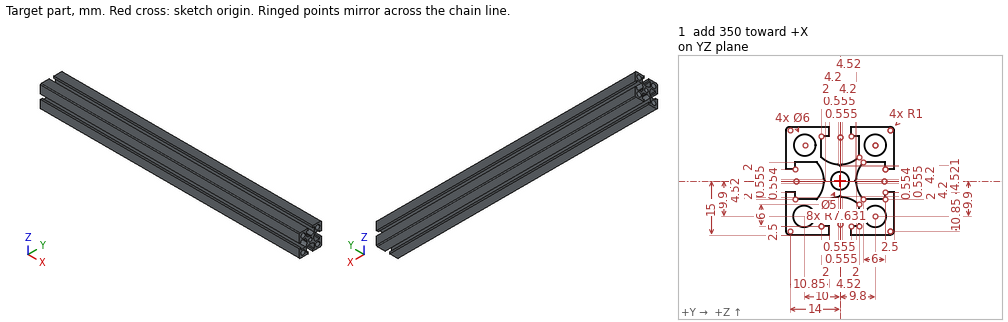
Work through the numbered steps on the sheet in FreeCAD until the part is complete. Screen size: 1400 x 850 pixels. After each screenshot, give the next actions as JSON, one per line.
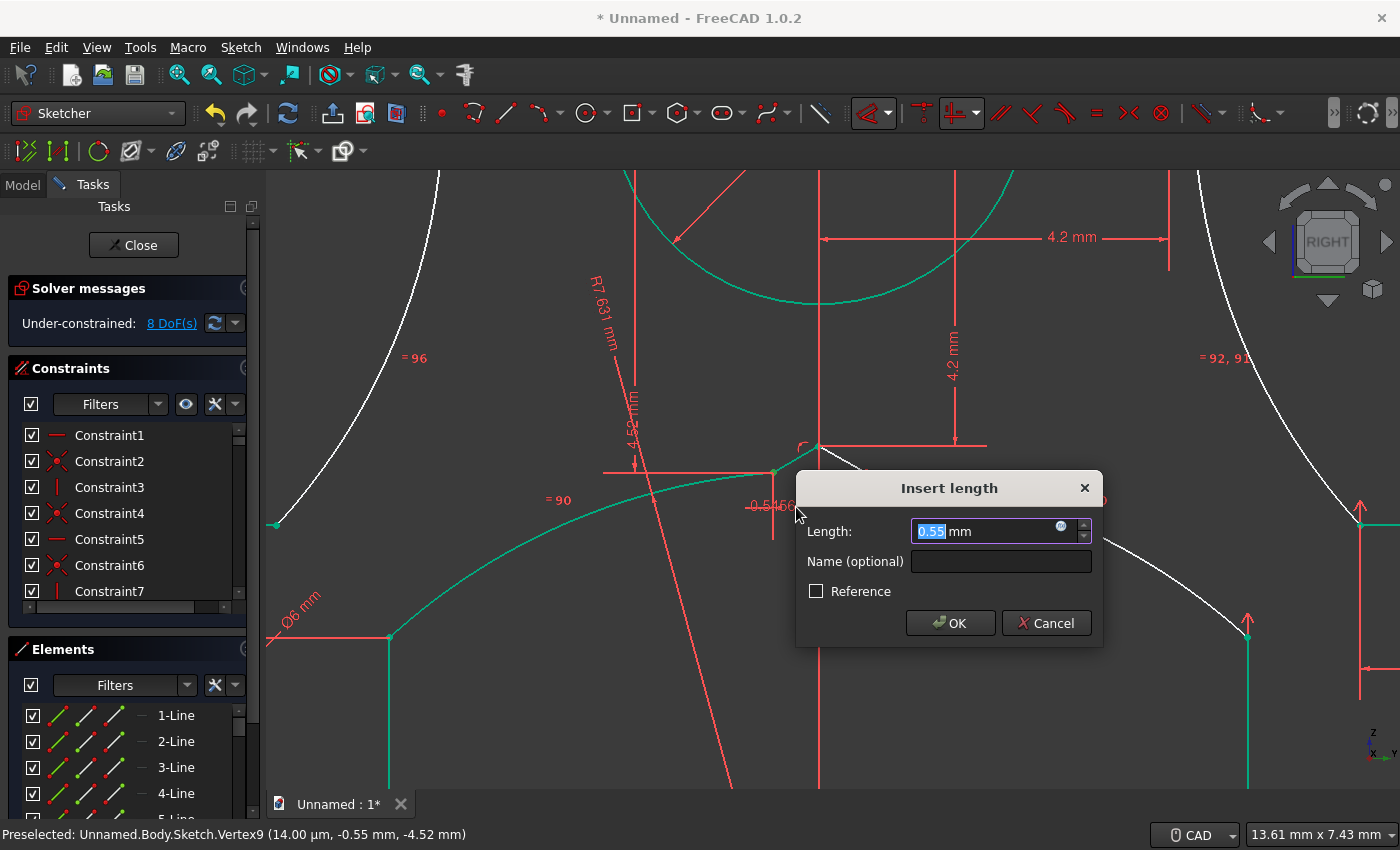
{"action": "type", "text": "0.555"}
{"action": "key", "text": "Return"}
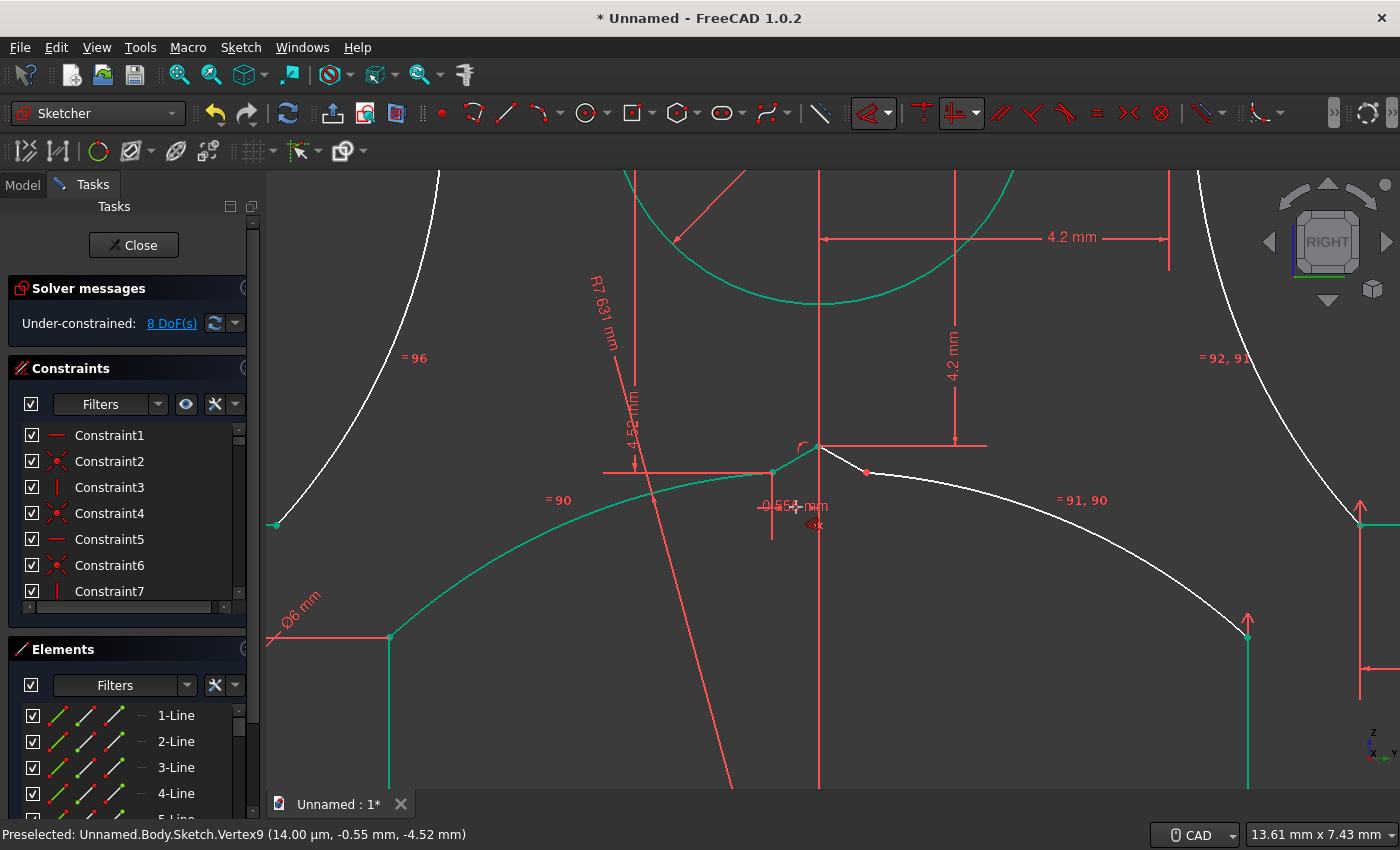
{"action": "left_click", "coordinate": [866, 473]}
{"action": "left_click", "coordinate": [842, 531]}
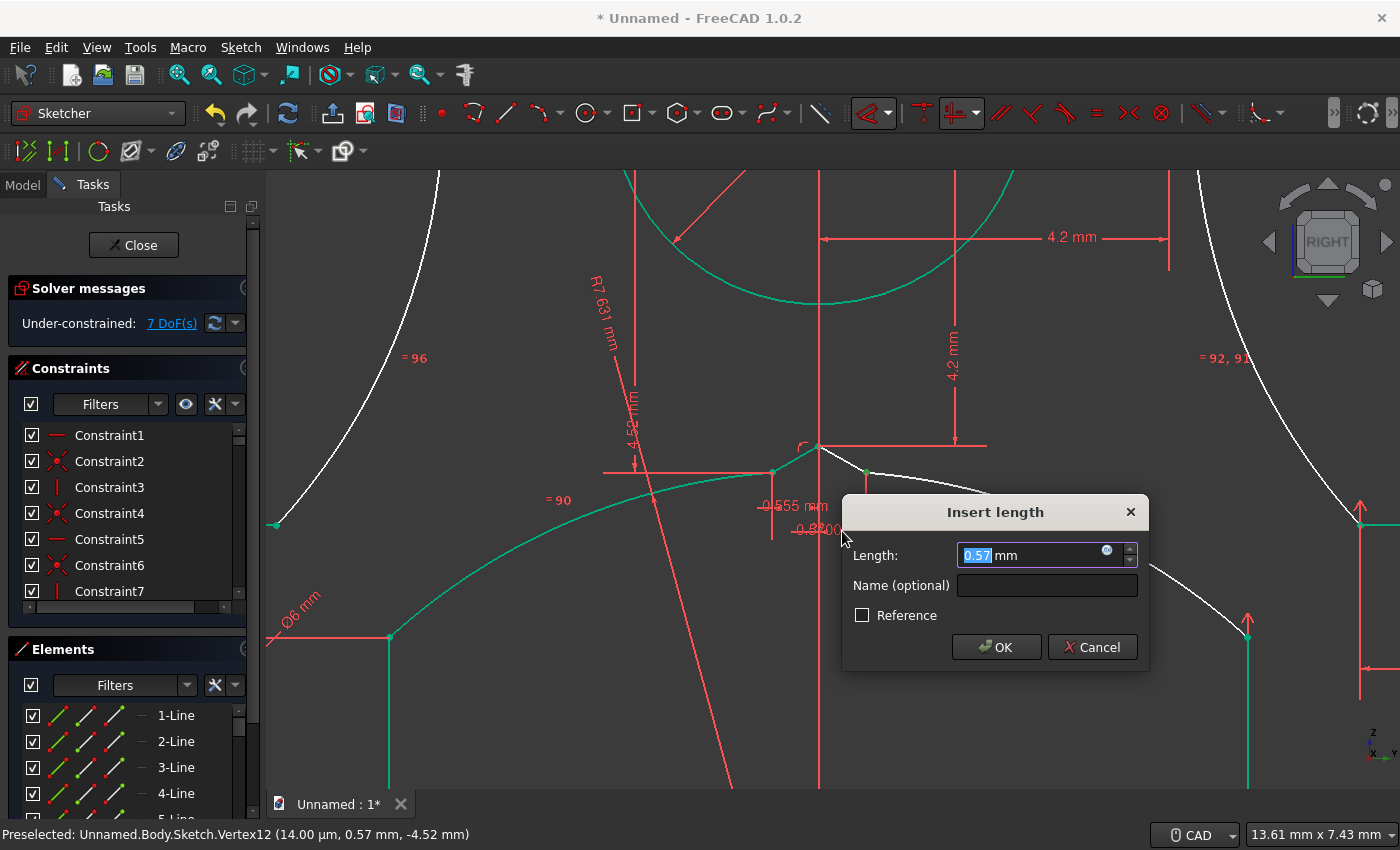
{"action": "type", "text": "0.555"}
{"action": "key", "text": "Return"}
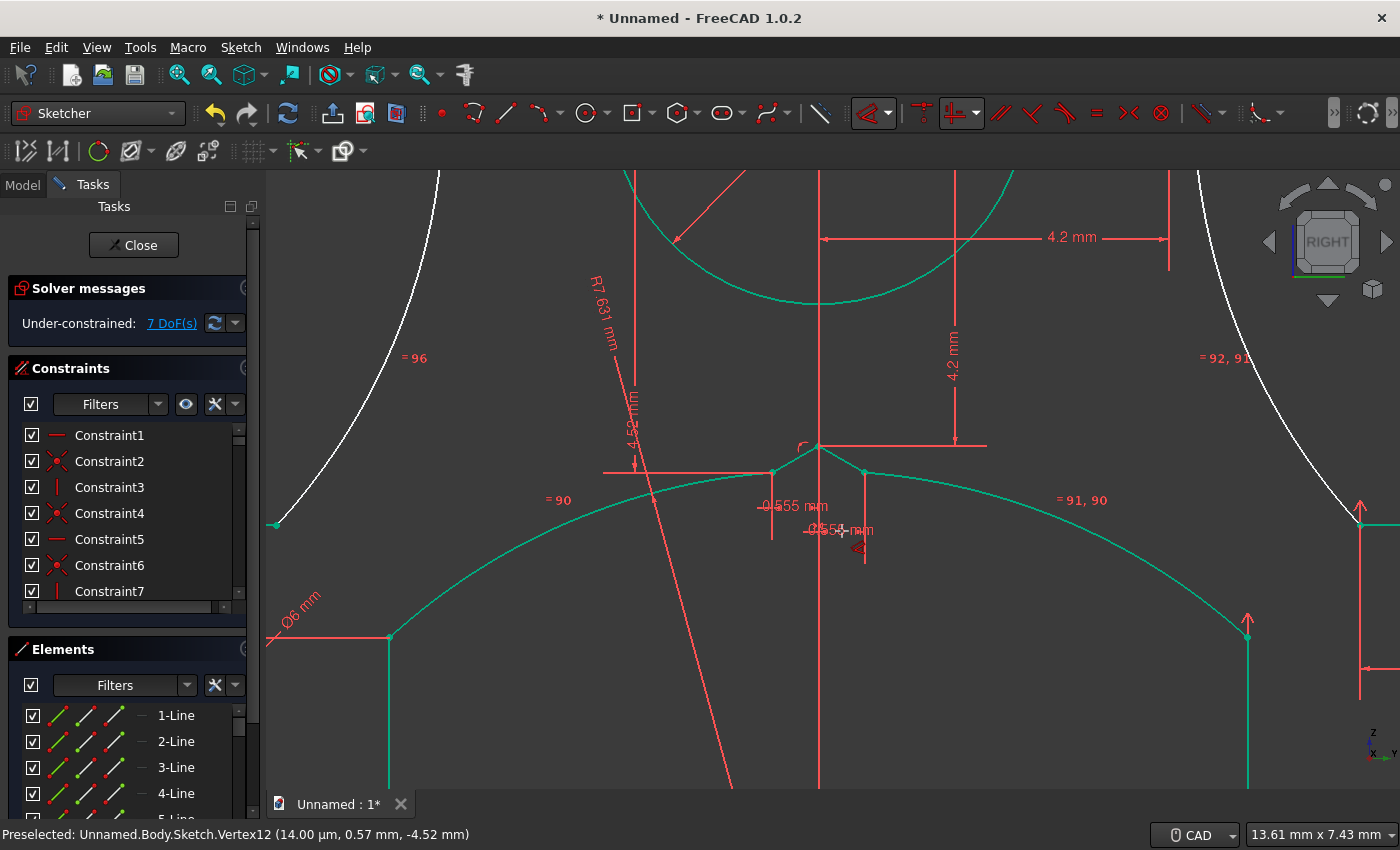
{"action": "scroll", "coordinate": [754, 555], "scroll_direction": "down", "scroll_amount": 9}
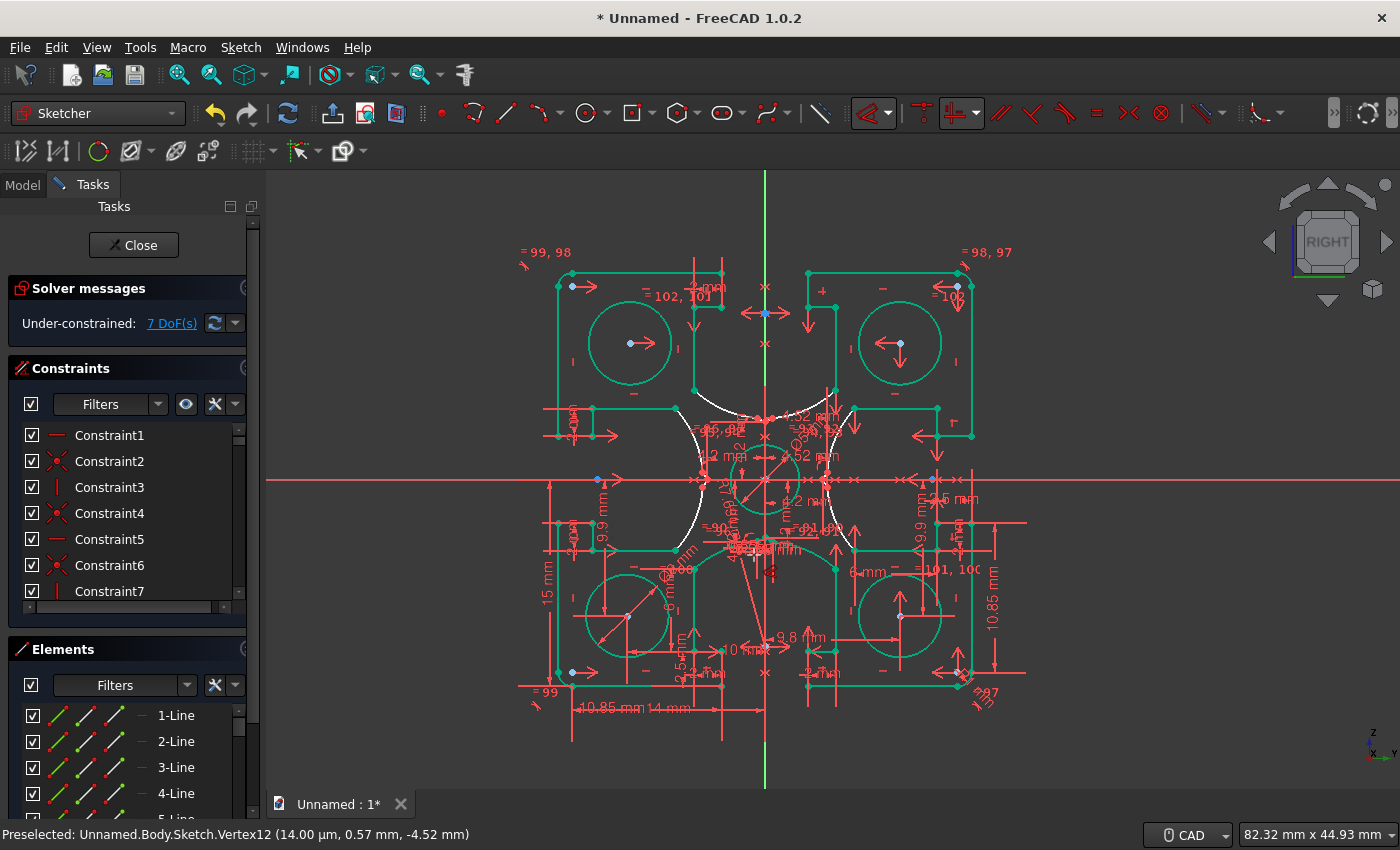
{"action": "scroll", "coordinate": [827, 488], "scroll_direction": "up", "scroll_amount": 9}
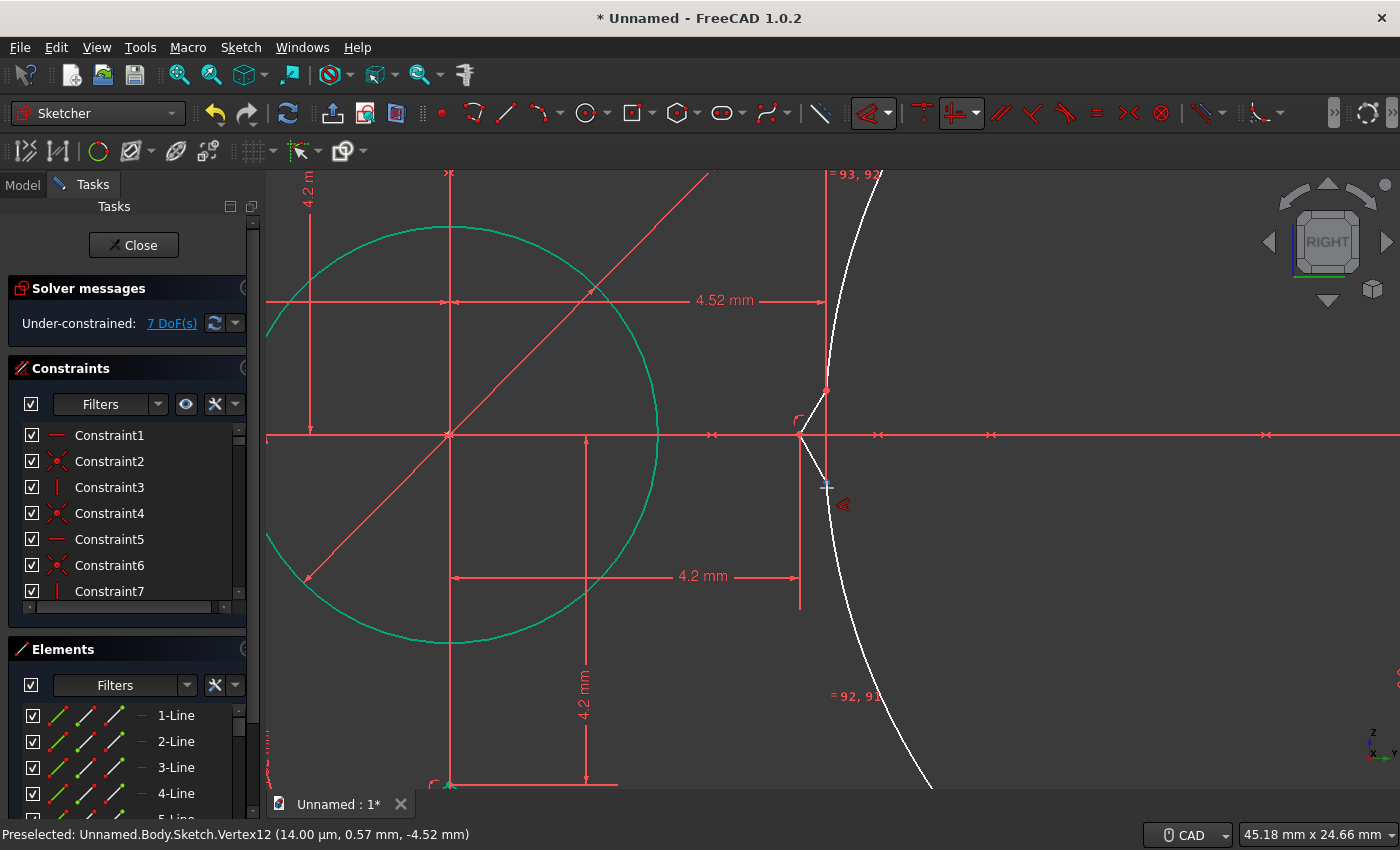
{"action": "left_click", "coordinate": [826, 482]}
{"action": "left_click", "coordinate": [860, 459]}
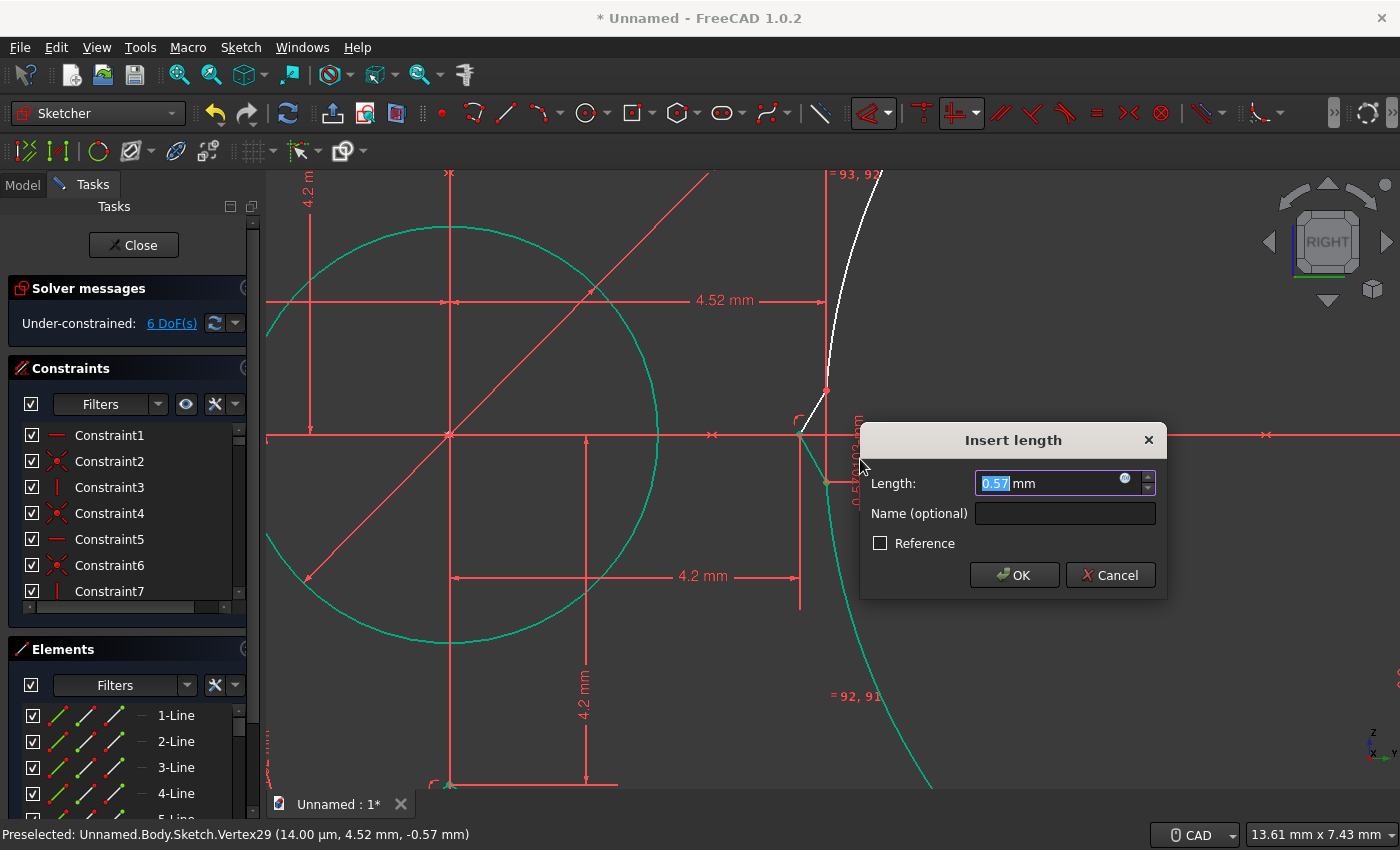
{"action": "type", "text": "0.554"}
{"action": "key", "text": "Return"}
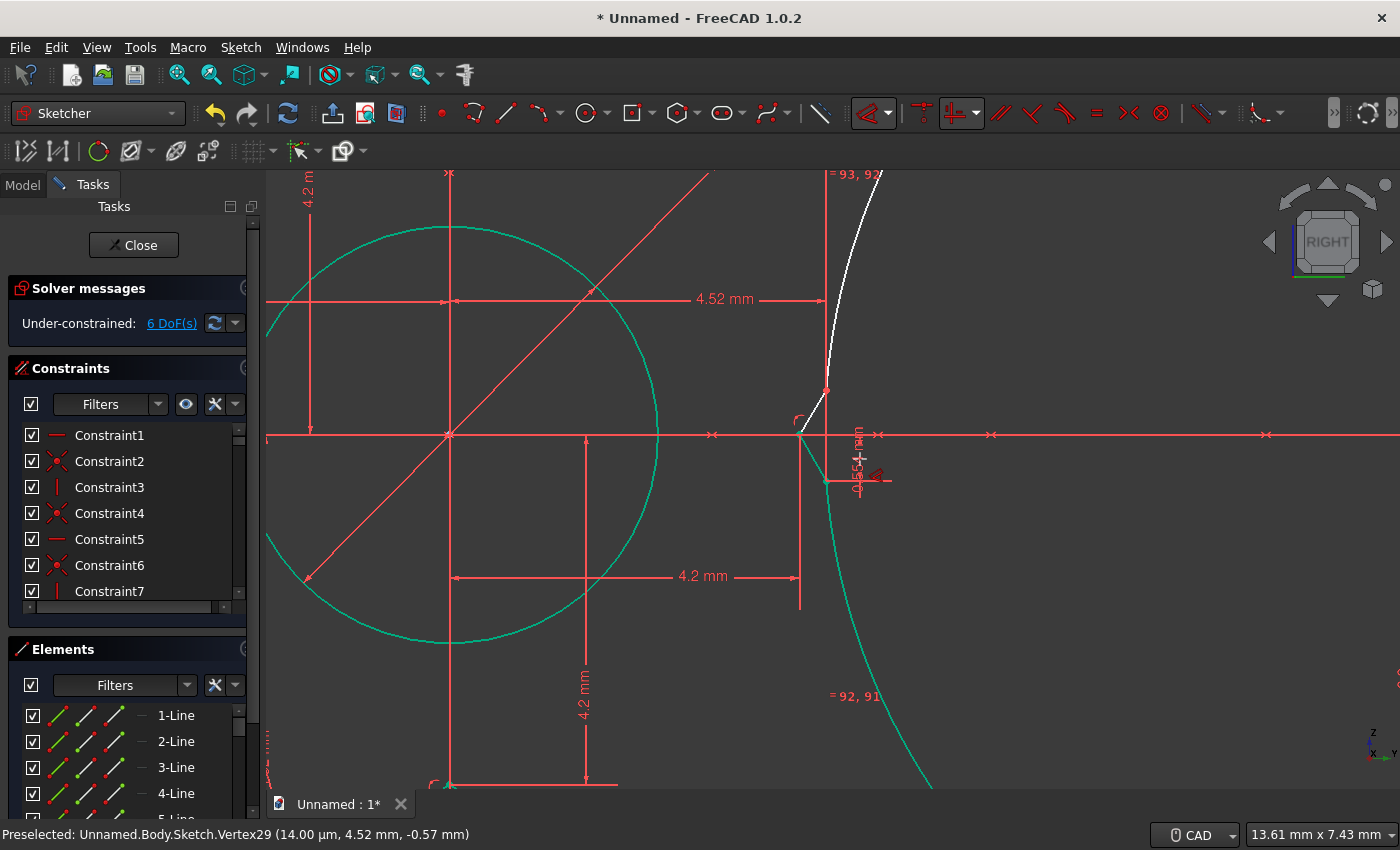
{"action": "left_click", "coordinate": [826, 390]}
{"action": "left_click", "coordinate": [860, 413]}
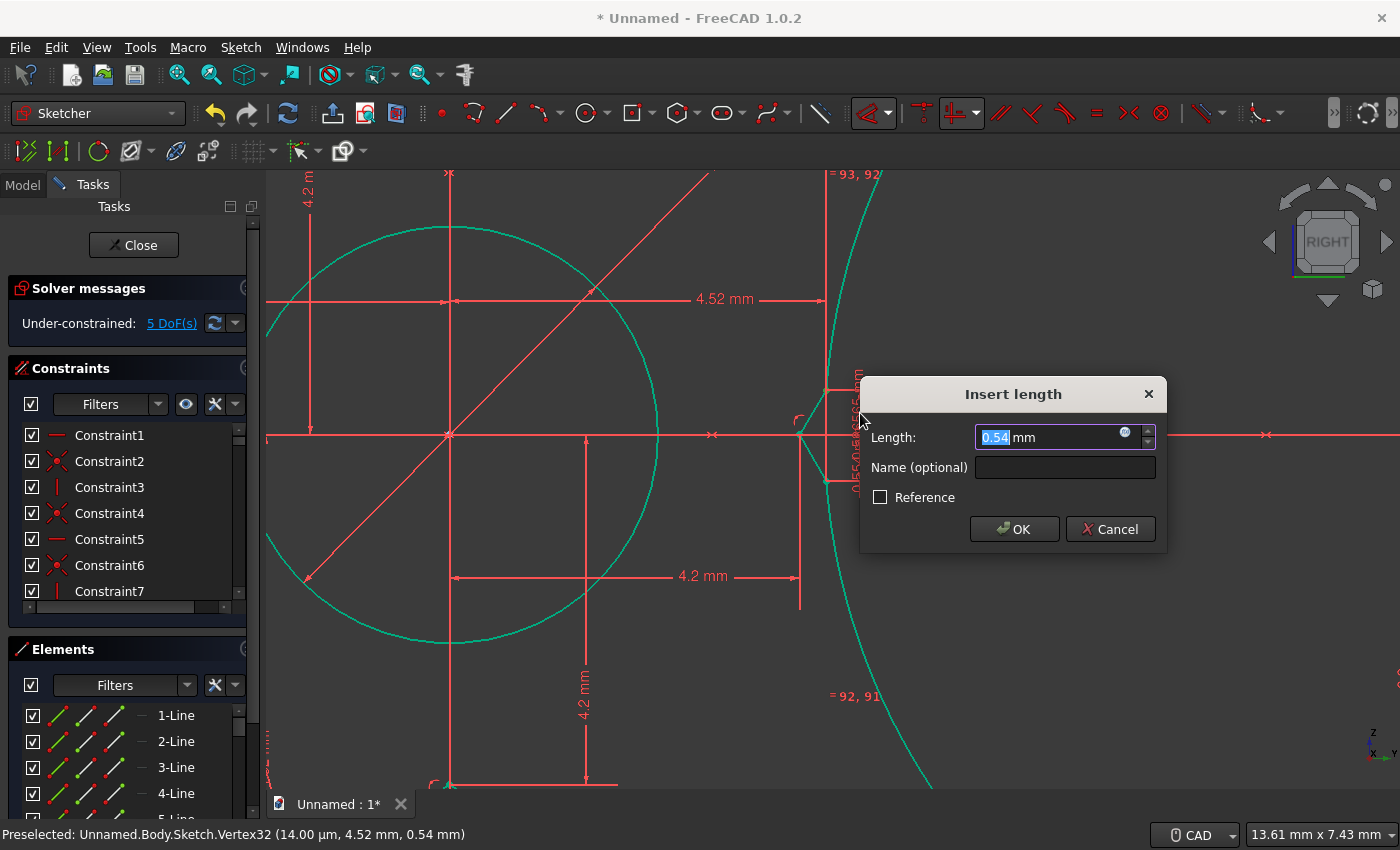
{"action": "type", "text": "0.555"}
{"action": "key", "text": "Return"}